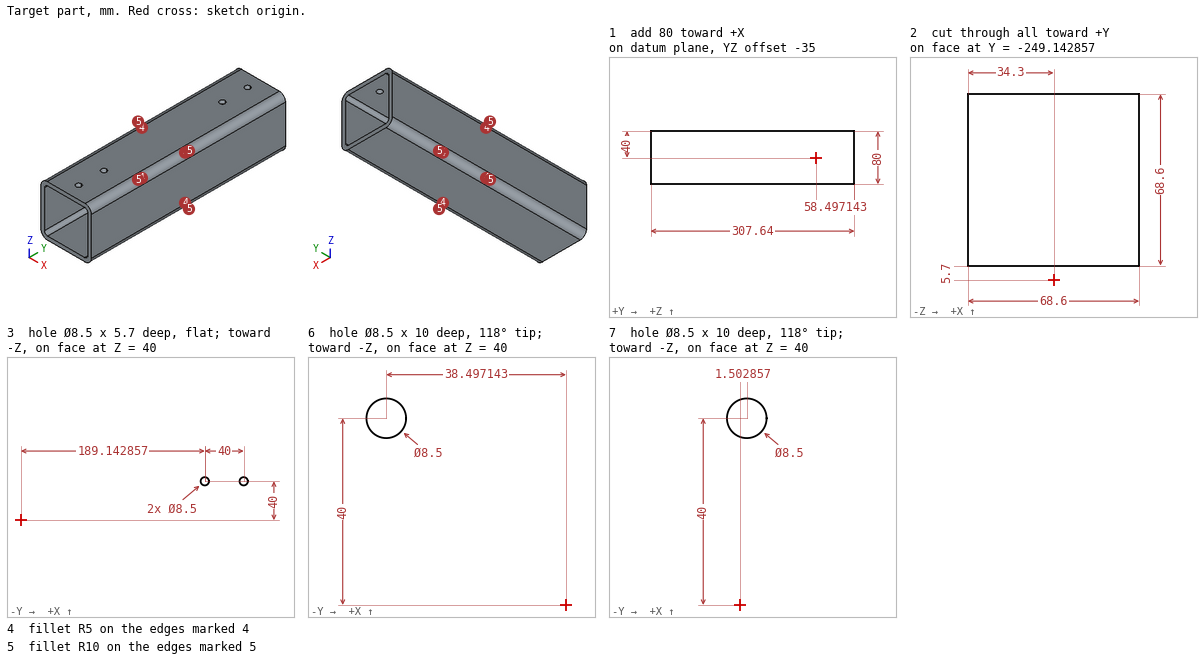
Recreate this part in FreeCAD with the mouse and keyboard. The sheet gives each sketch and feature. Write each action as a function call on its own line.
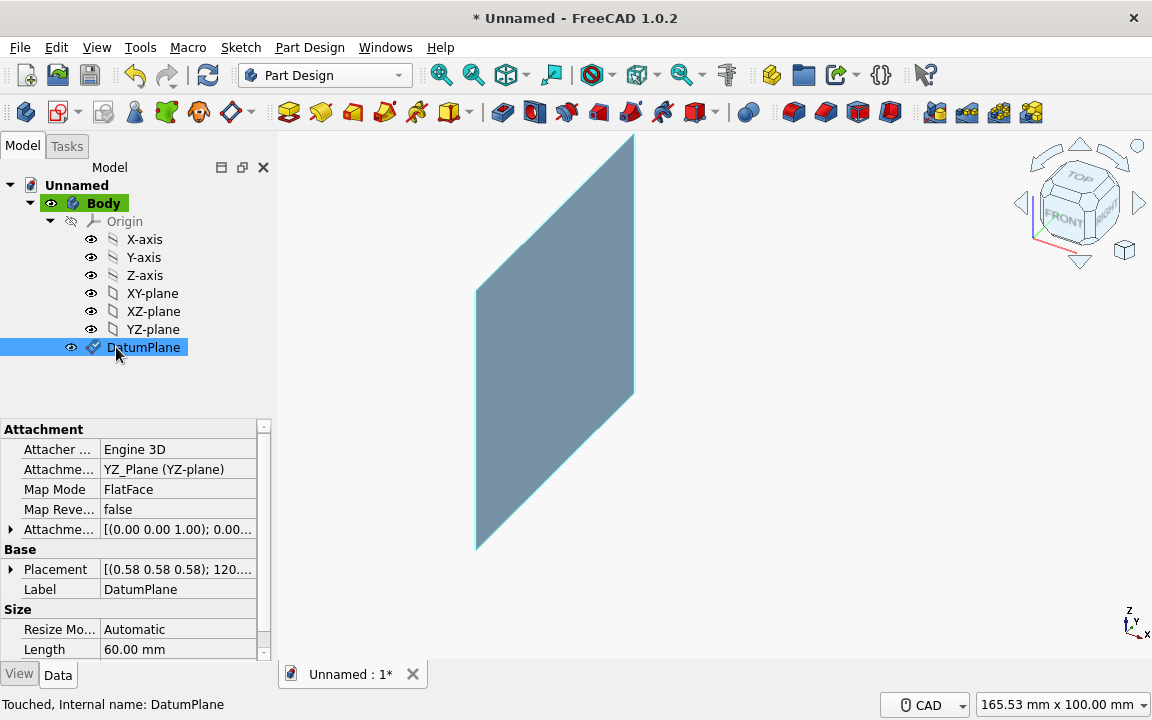
click(58, 112)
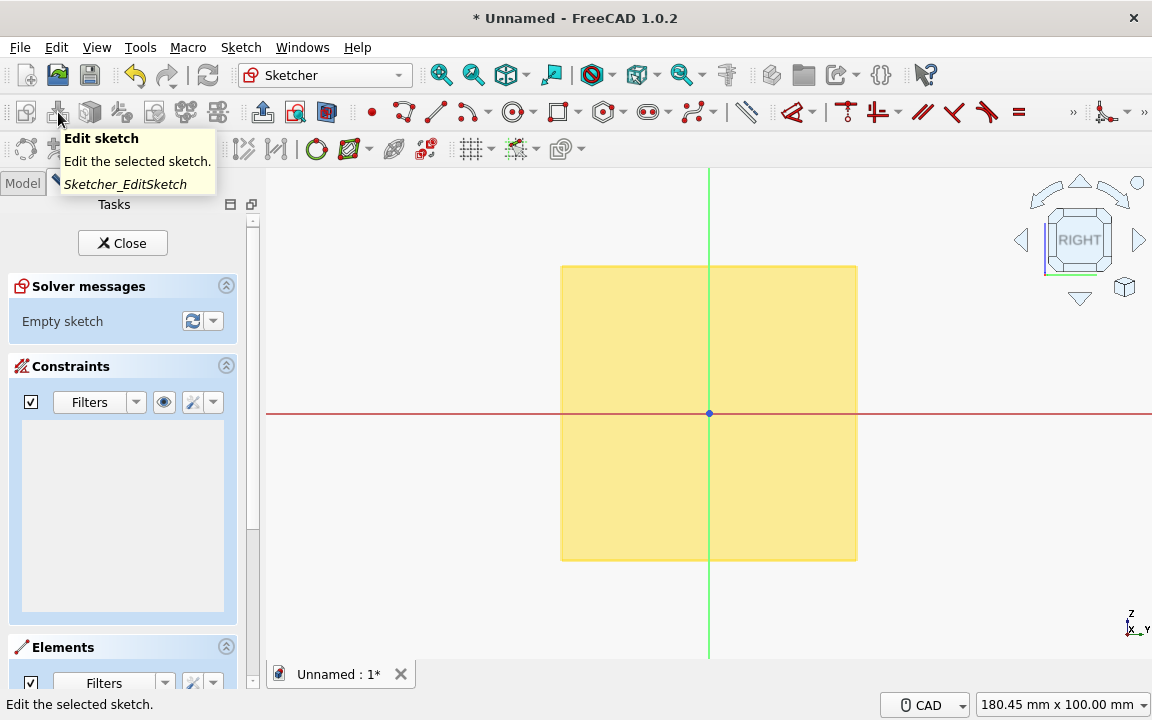
scroll(813, 413, down, 6)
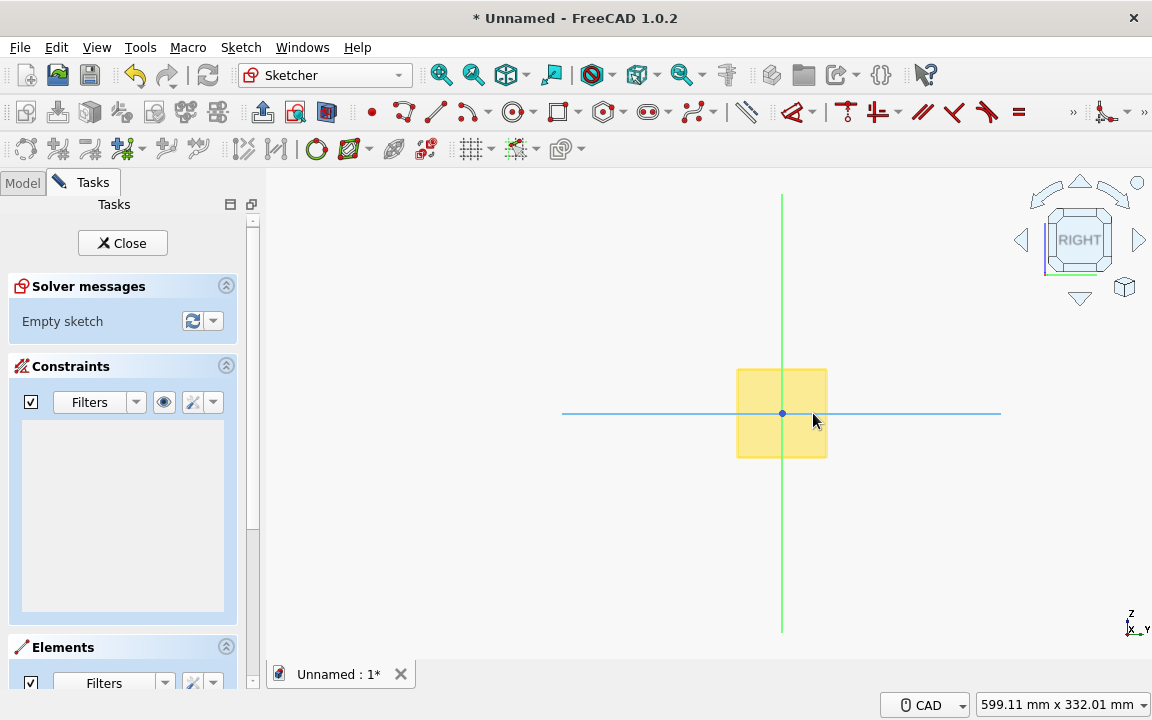
key(g)
key(r)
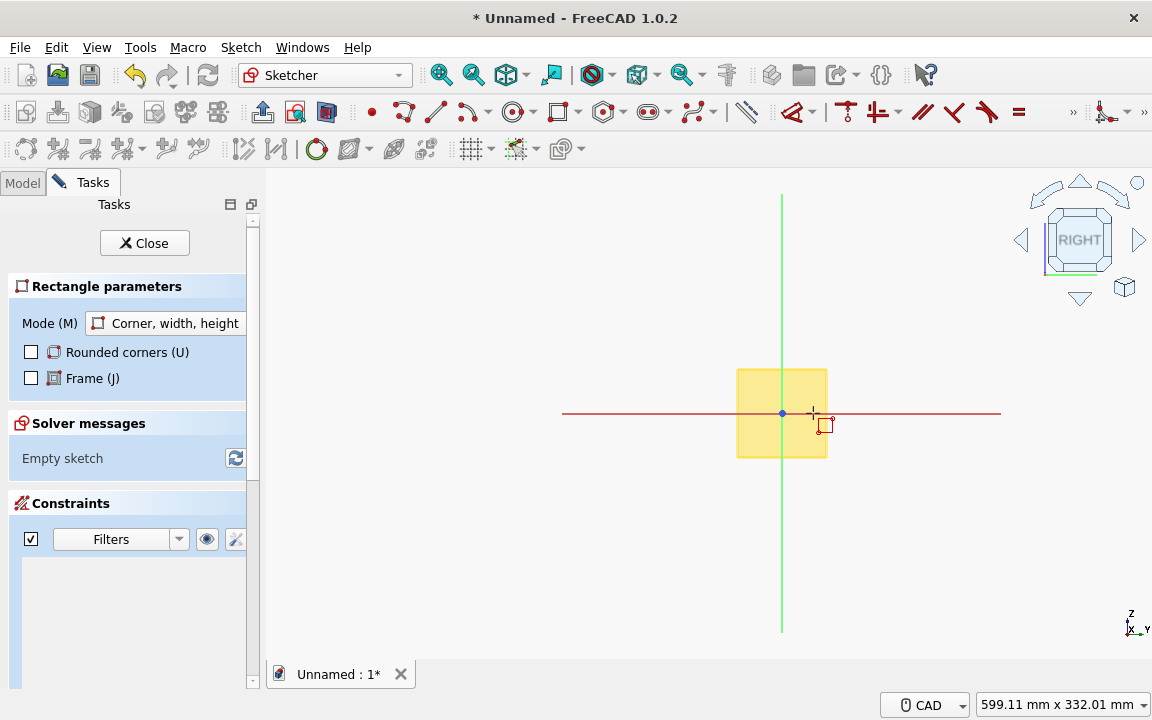
click(414, 354)
move(869, 473)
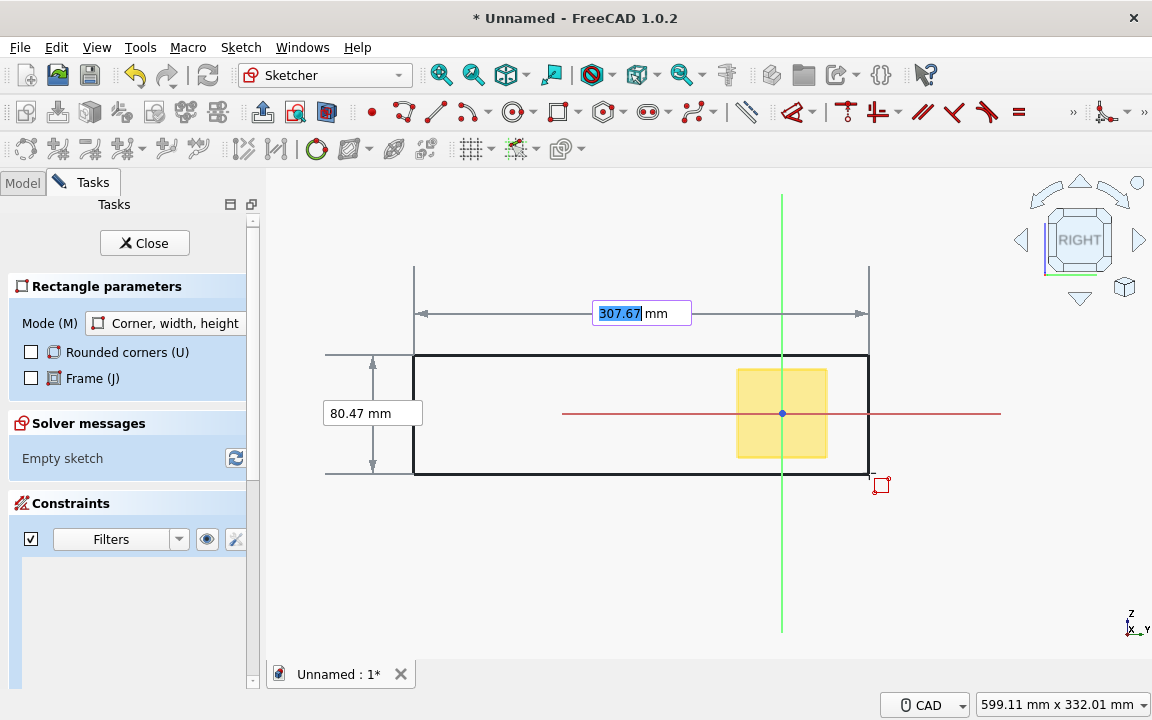
text(307.64)
key(Tab)
text(80)
key(Return)
key(Escape)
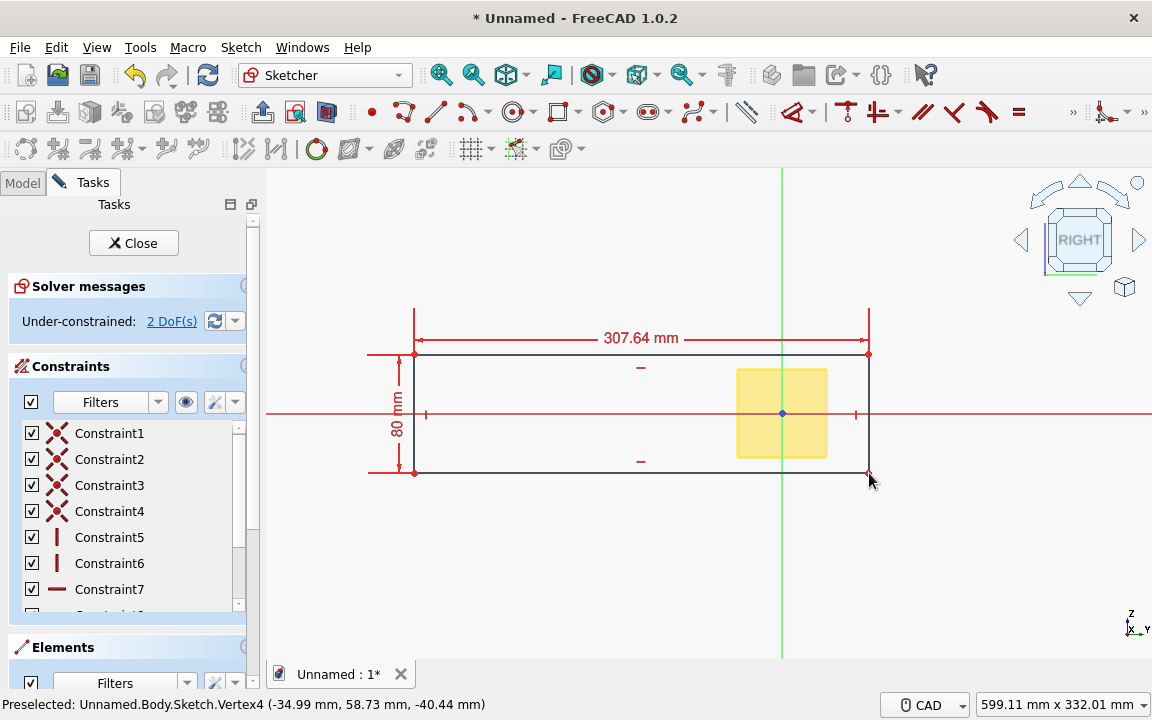
click(414, 355)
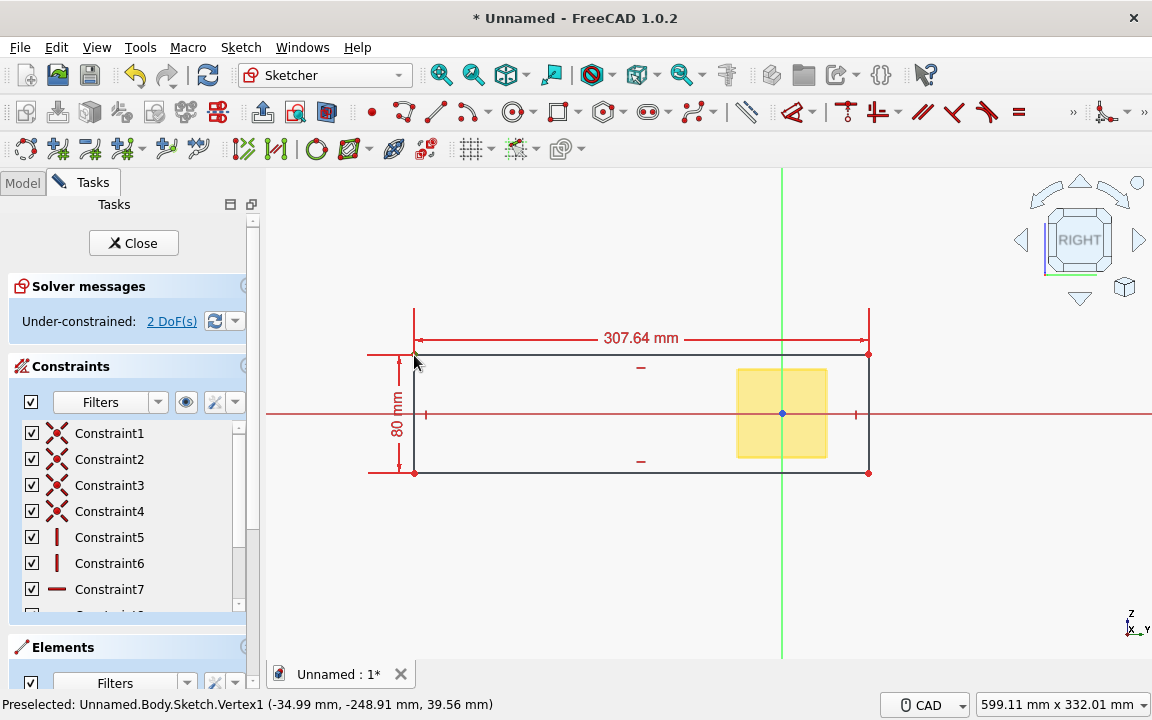
key(i)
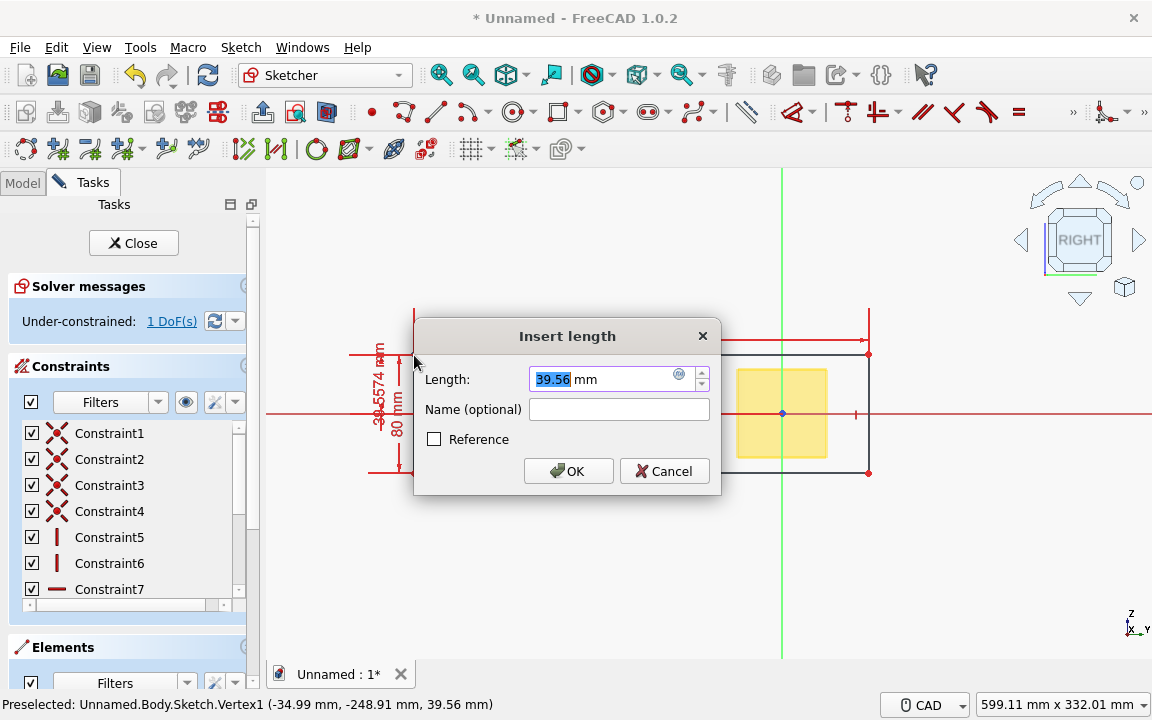
text(40)
key(Return)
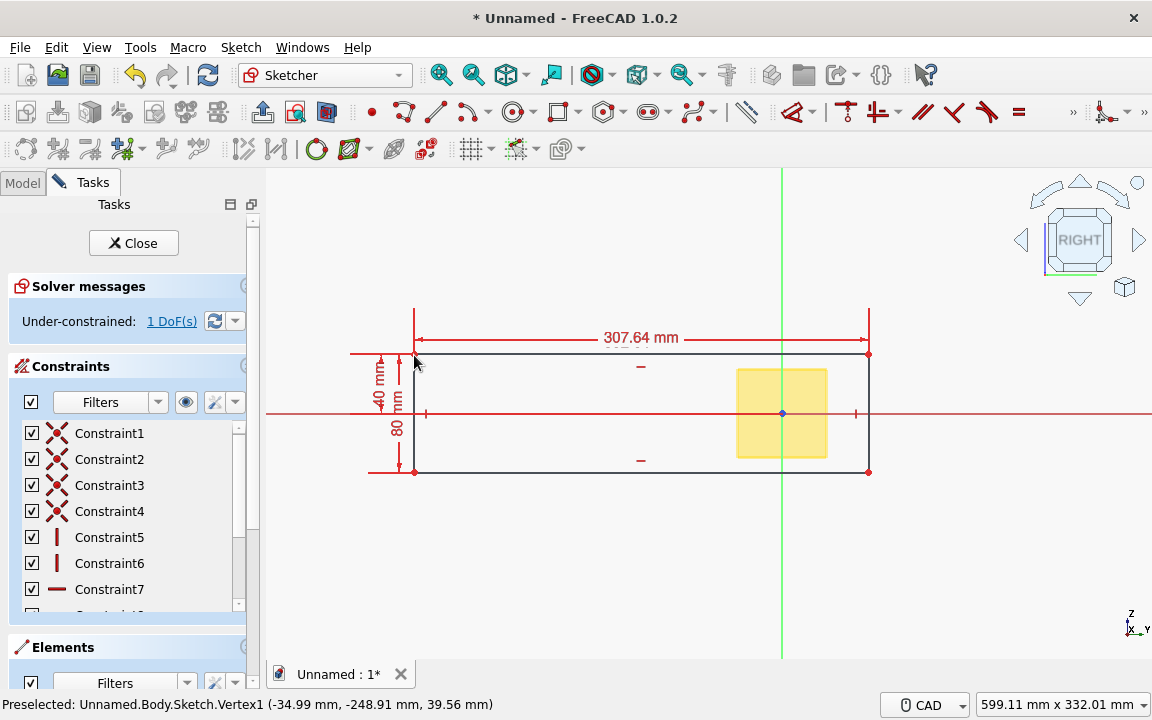
click(869, 473)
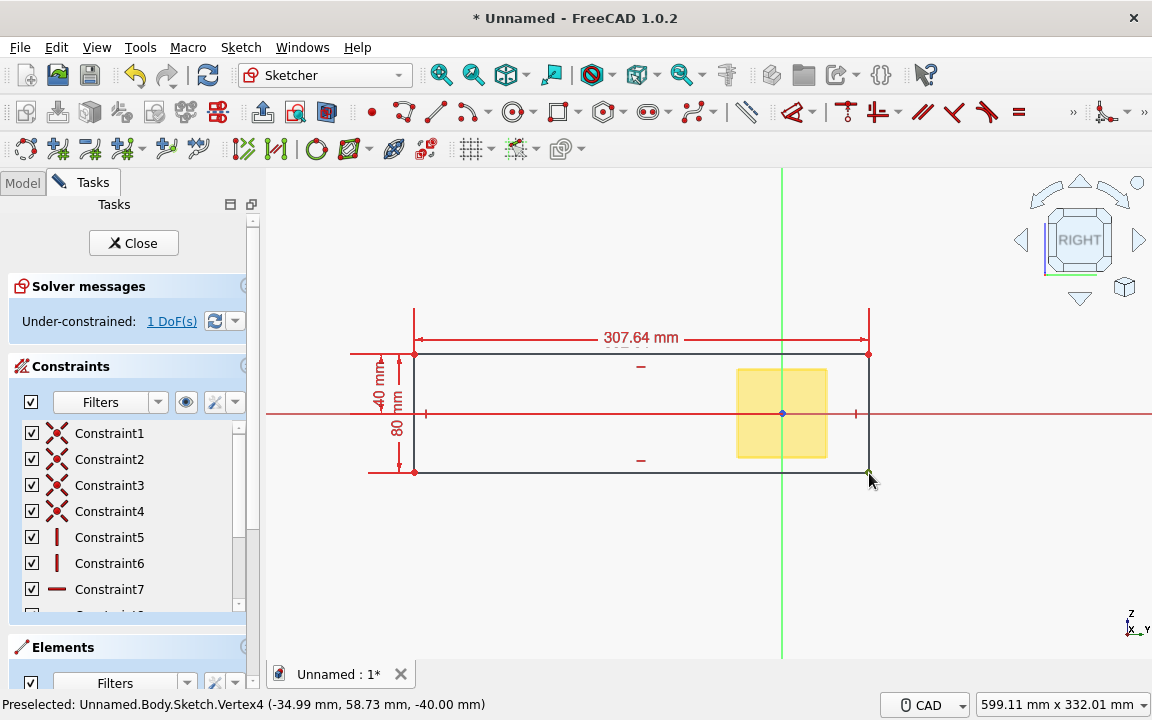
key(l)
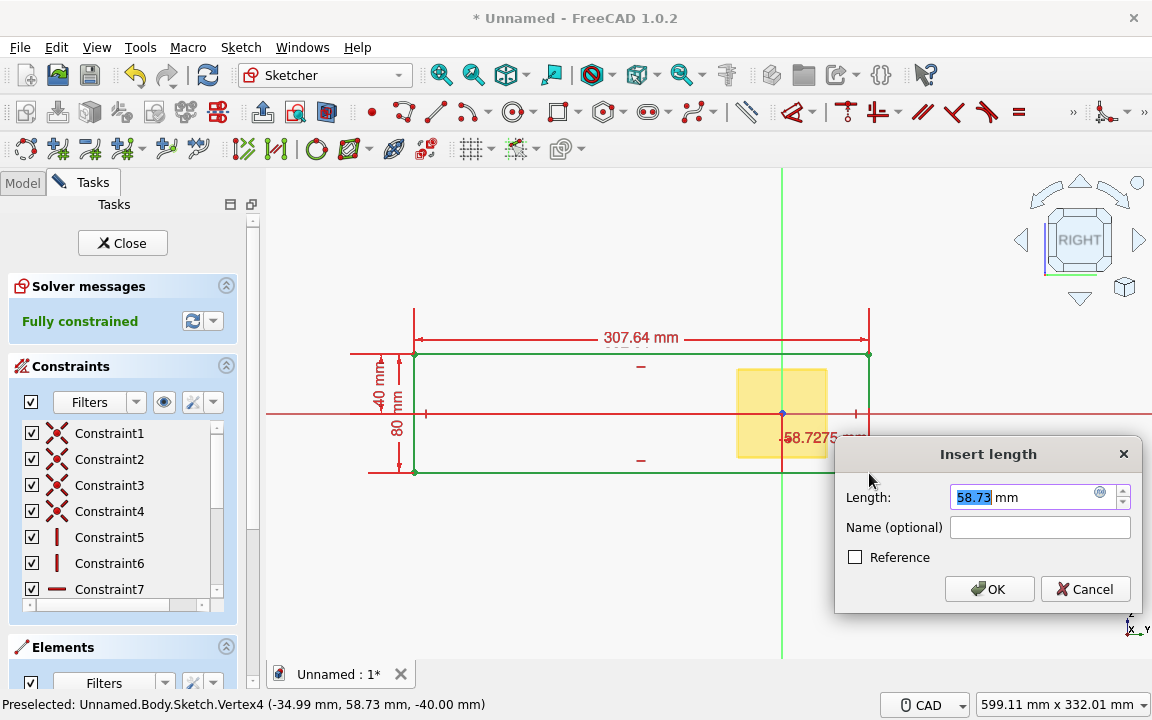
text(58.497143)
key(Return)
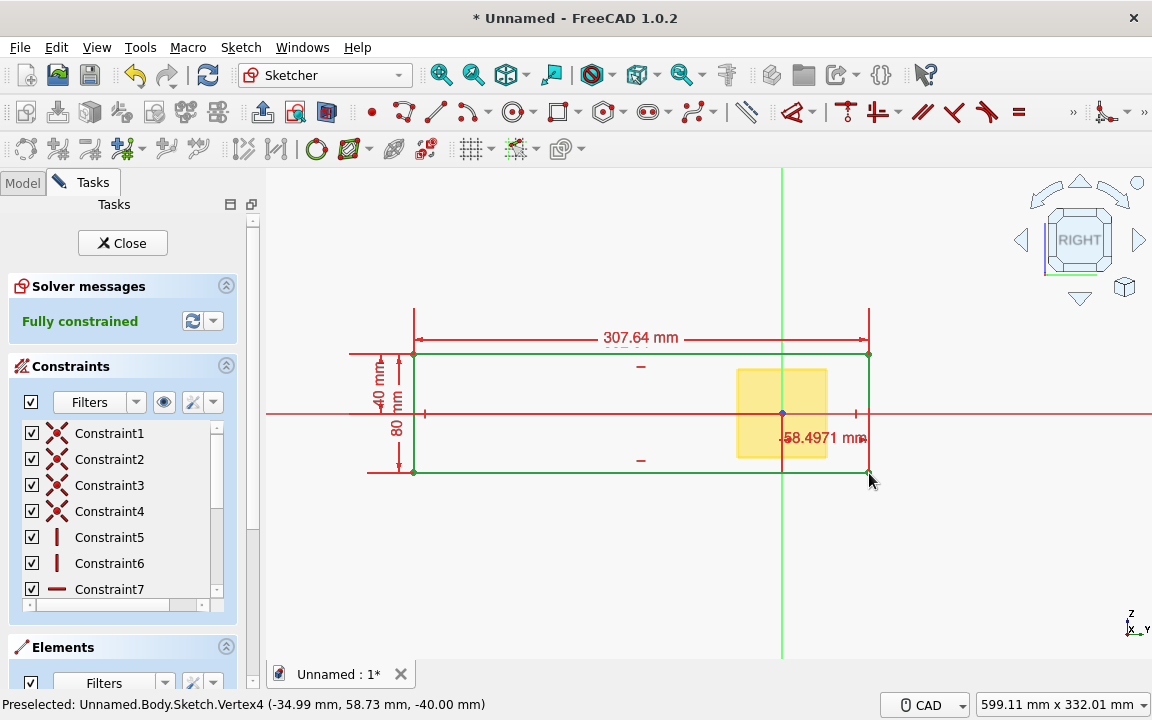
click(123, 243)